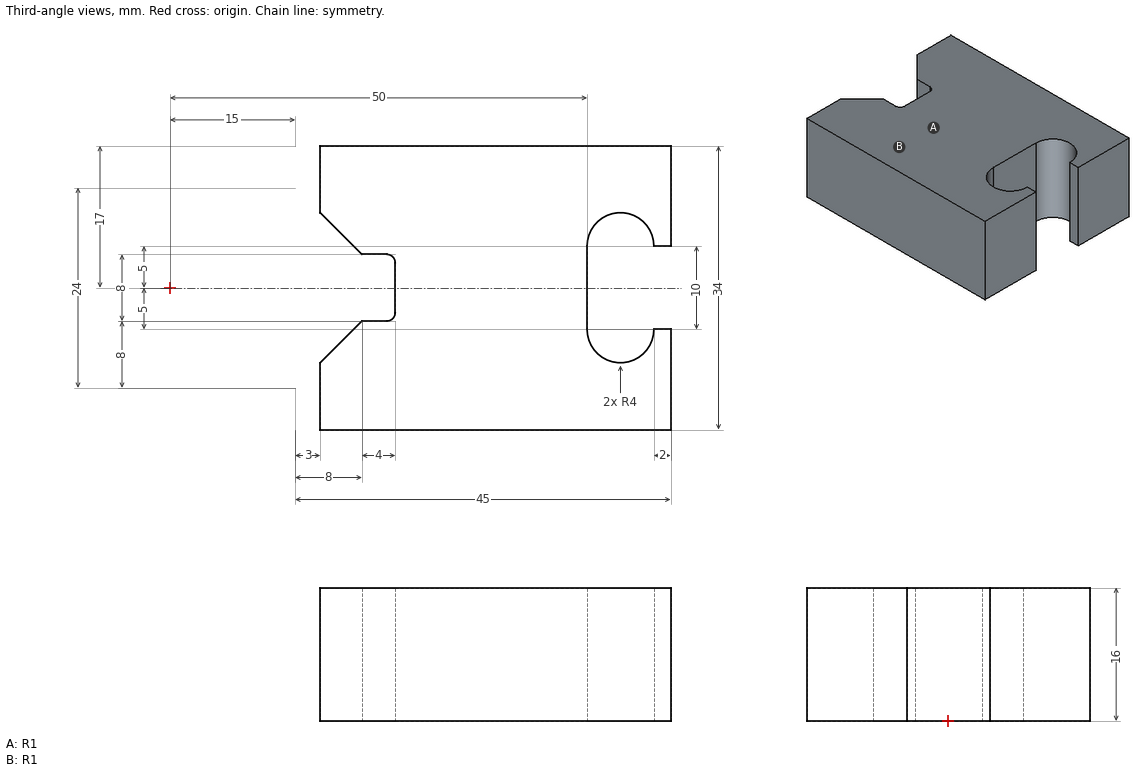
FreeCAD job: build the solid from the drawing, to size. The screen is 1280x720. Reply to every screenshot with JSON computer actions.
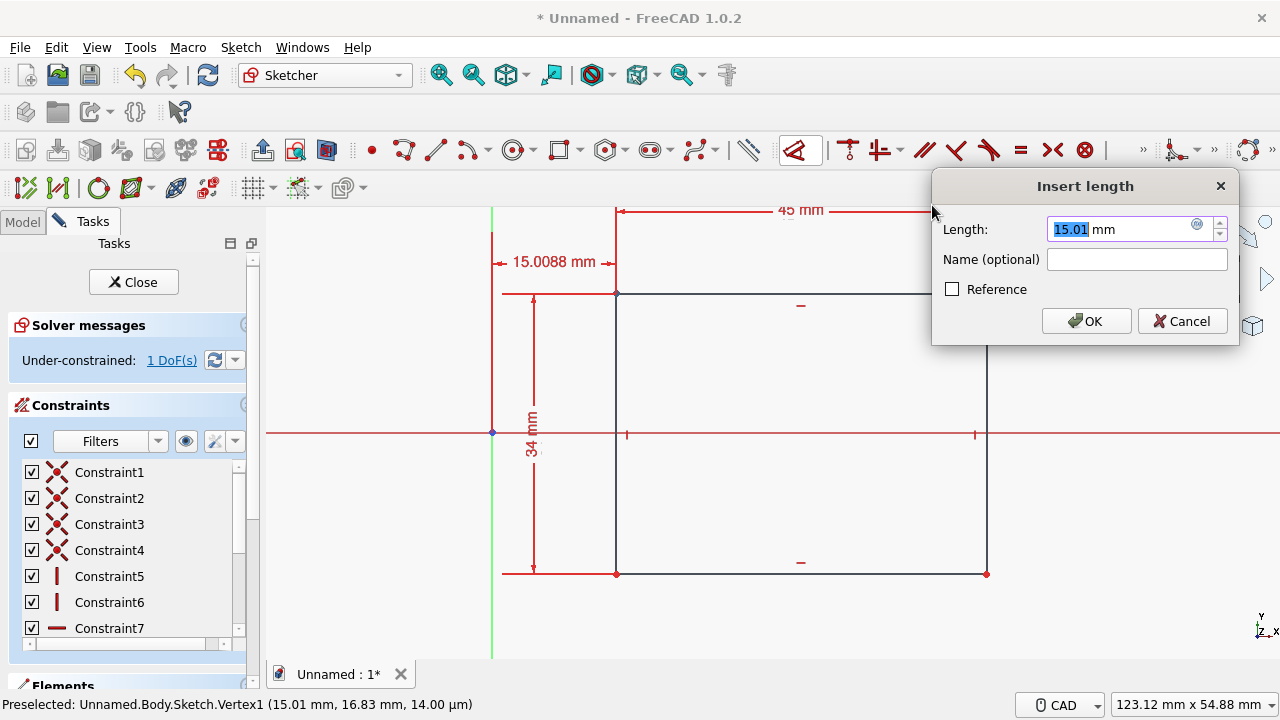
{"action": "type", "text": "15"}
{"action": "key", "text": "Return"}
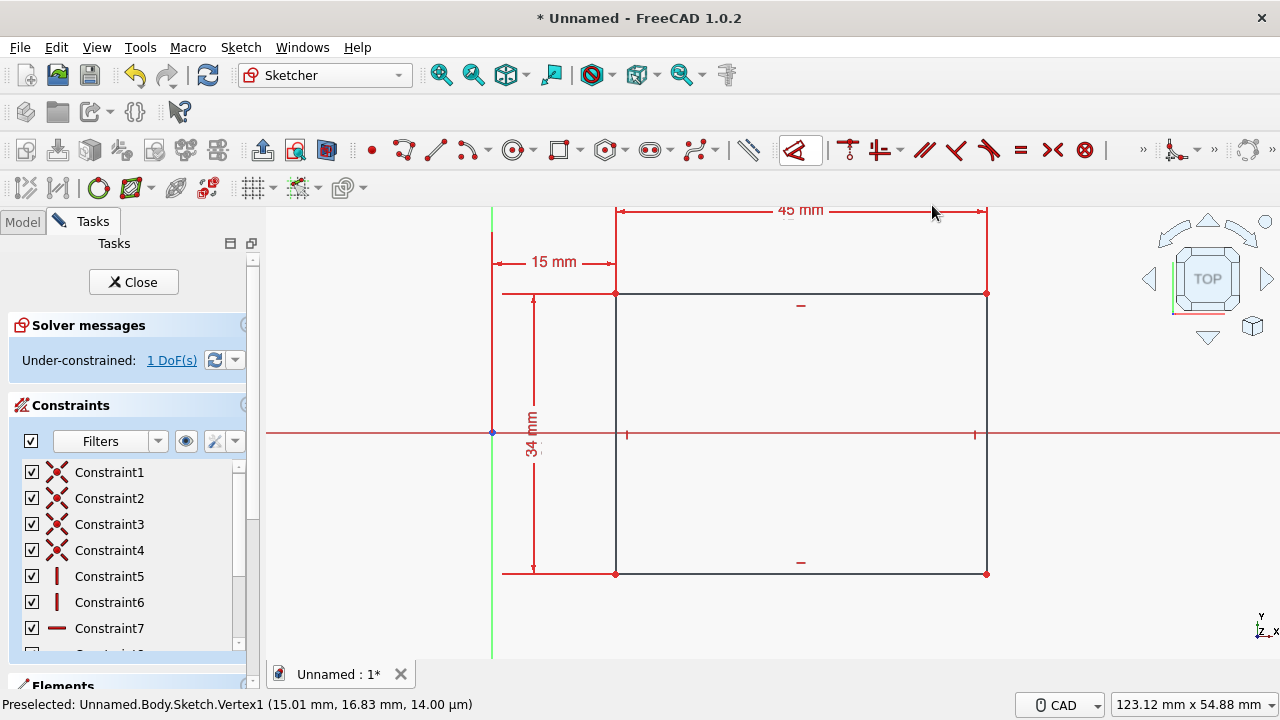
{"action": "left_click", "coordinate": [616, 294]}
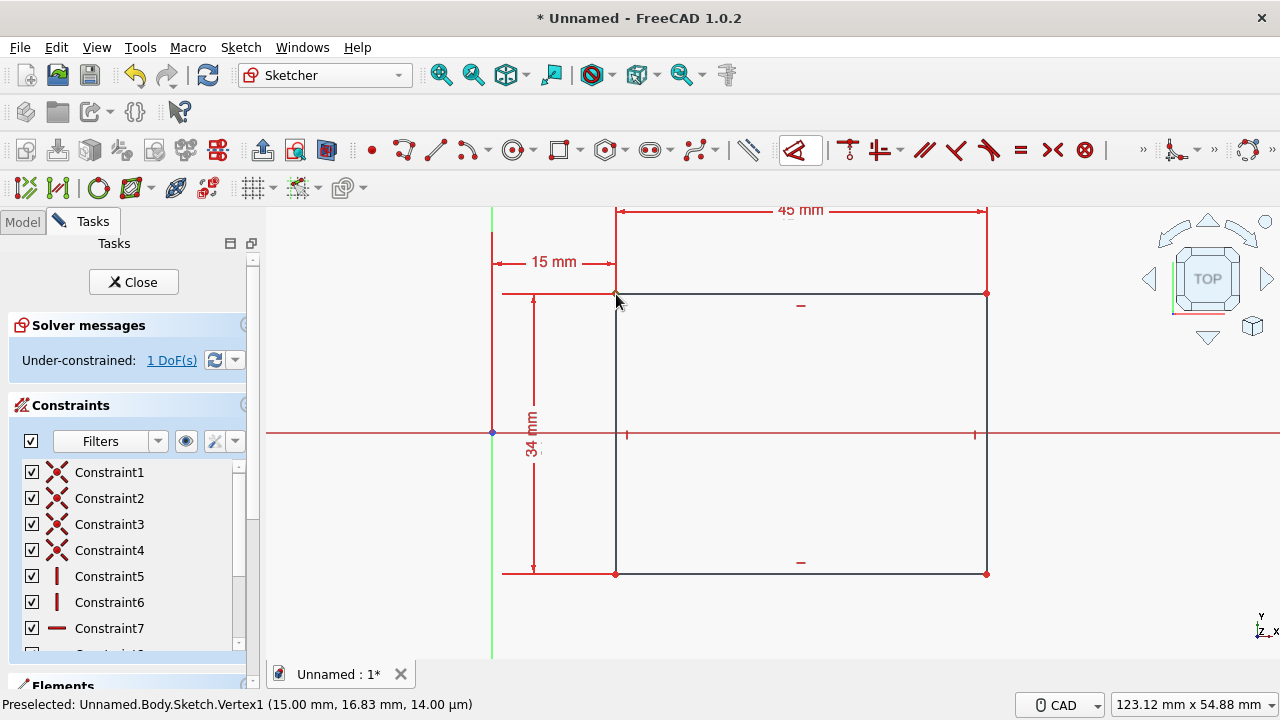
{"action": "left_click", "coordinate": [816, 150]}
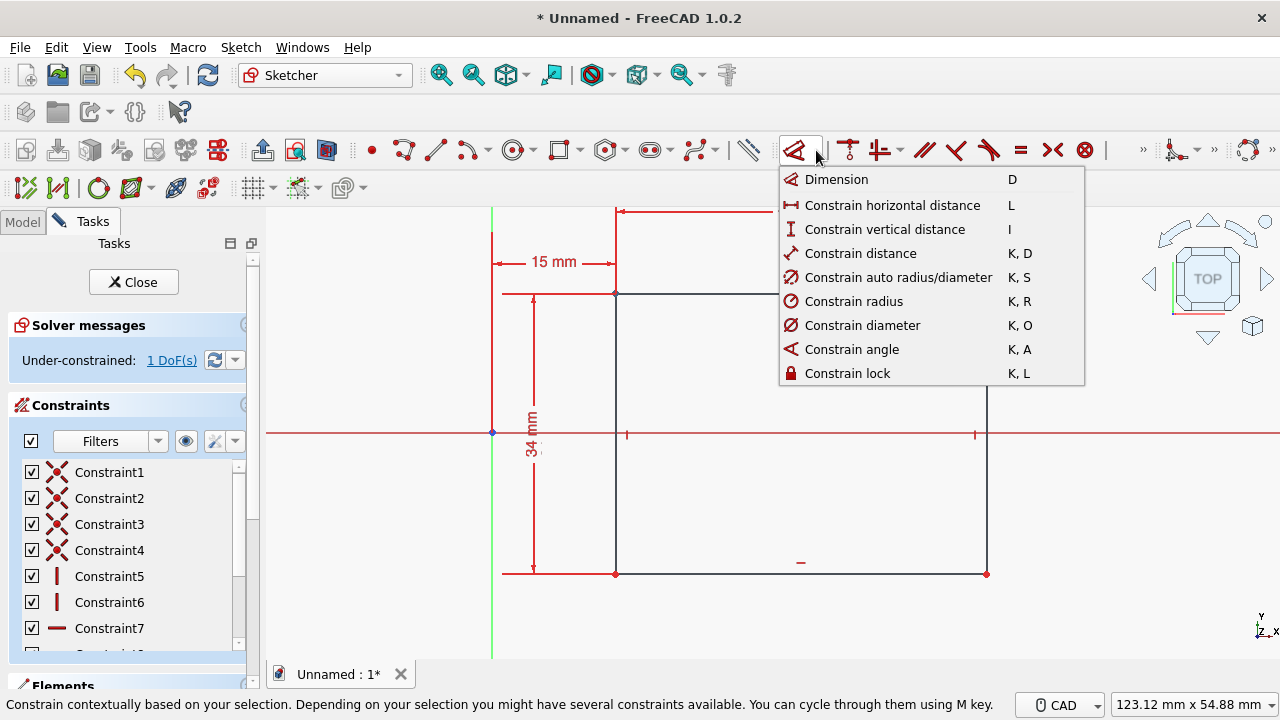
{"action": "left_click", "coordinate": [932, 229]}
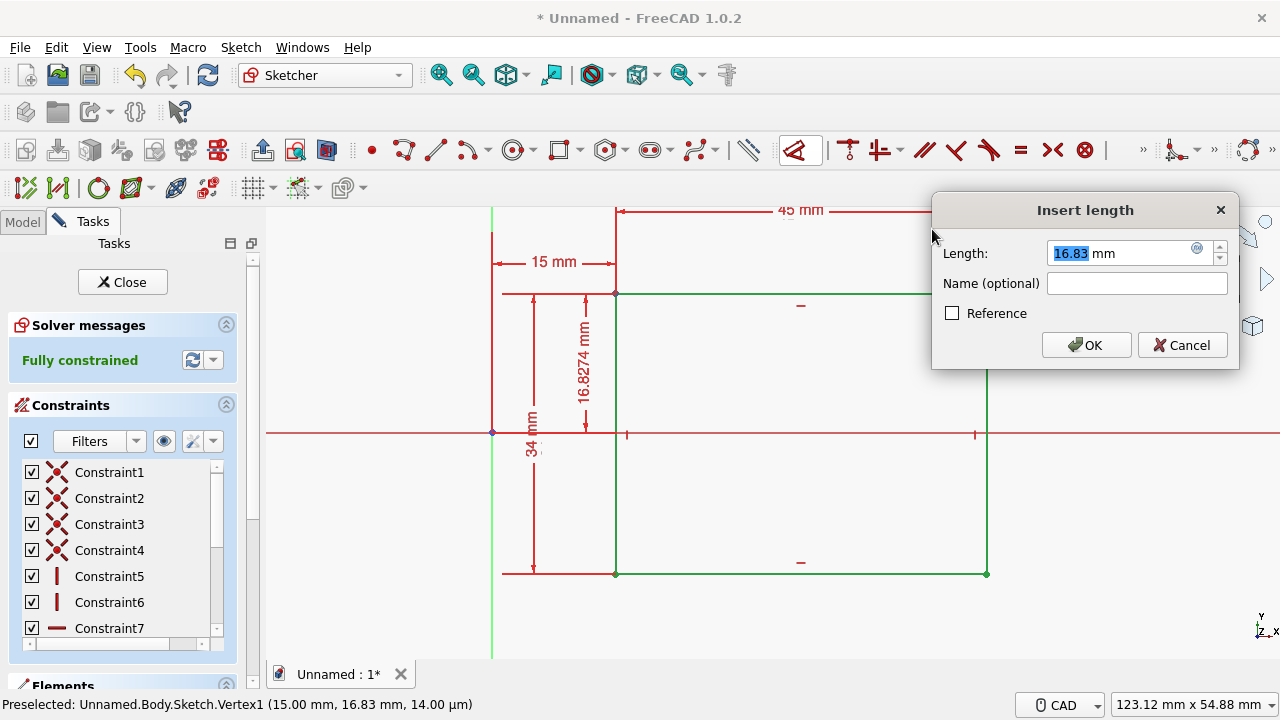
{"action": "type", "text": "17"}
{"action": "key", "text": "Return"}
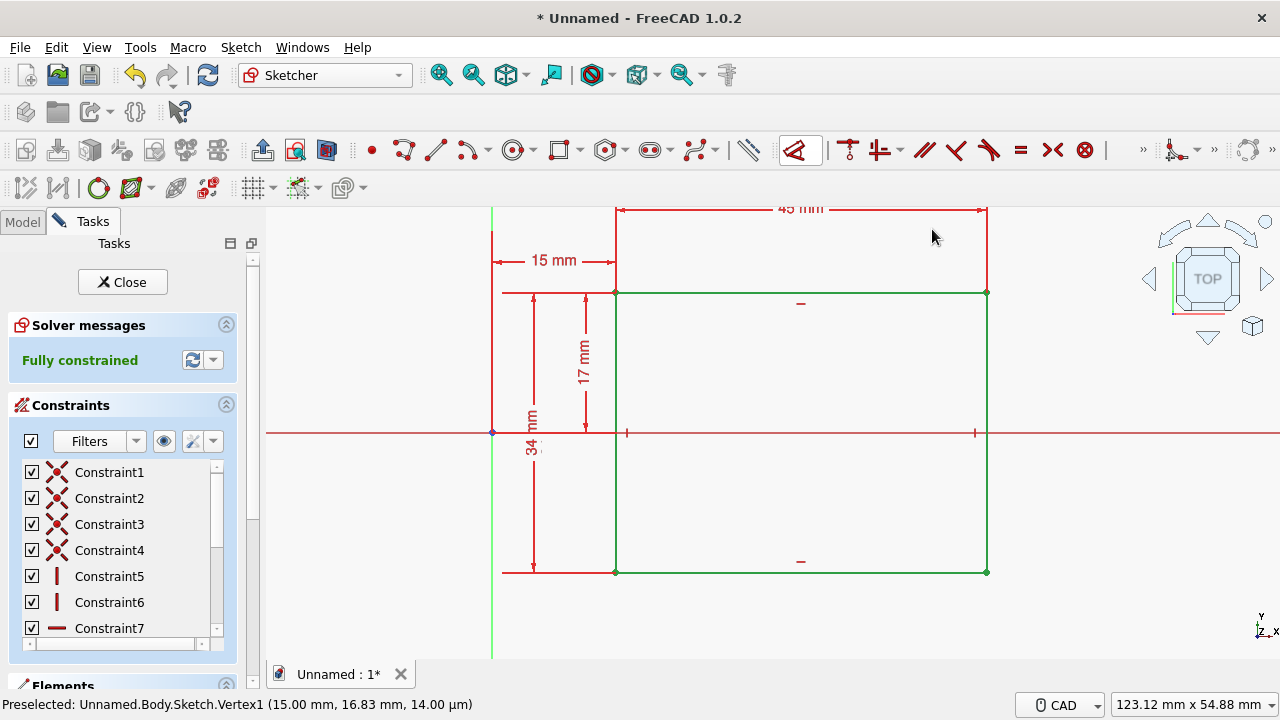
{"action": "left_click", "coordinate": [123, 282]}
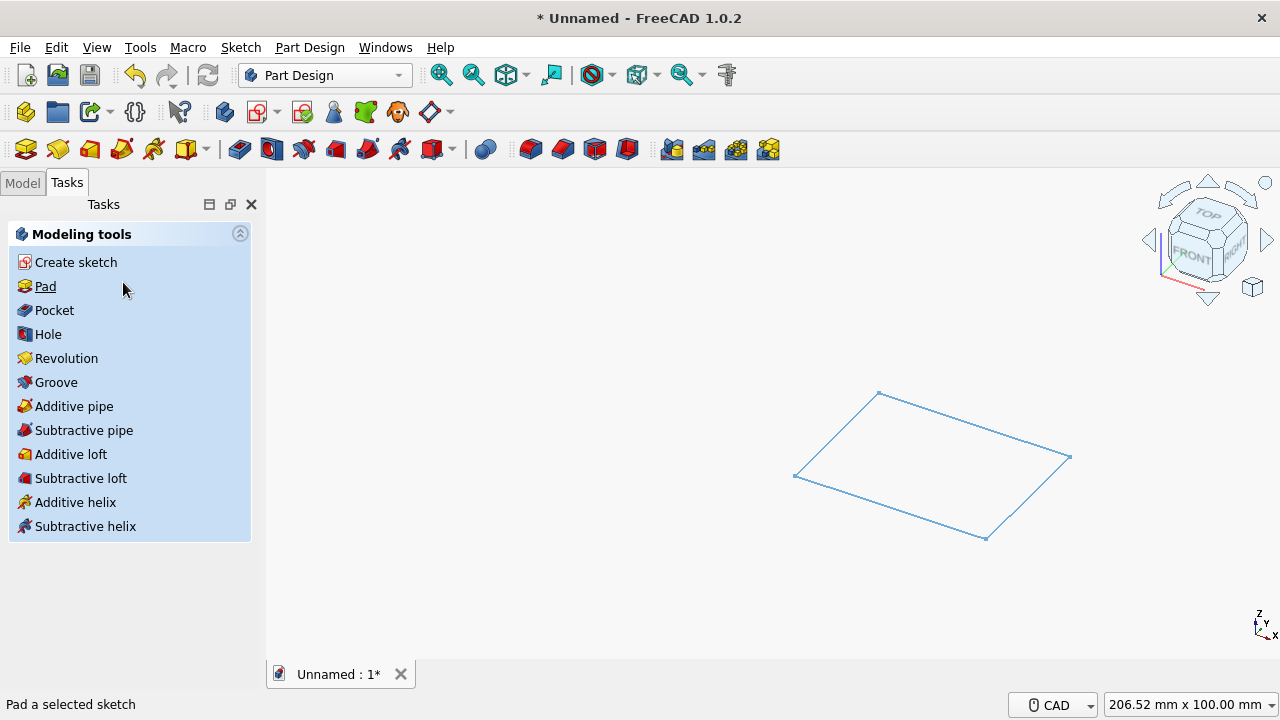
{"action": "left_click", "coordinate": [26, 150]}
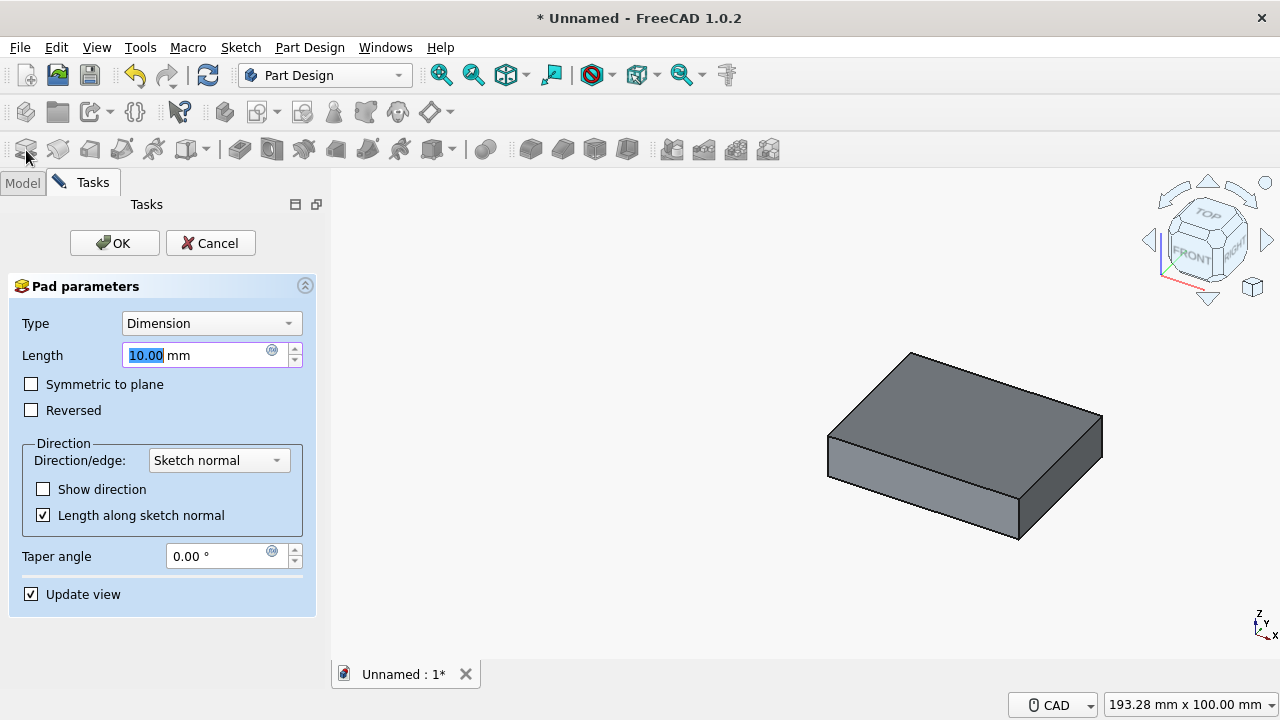
{"action": "type", "text": "16"}
{"action": "key", "text": "Tab"}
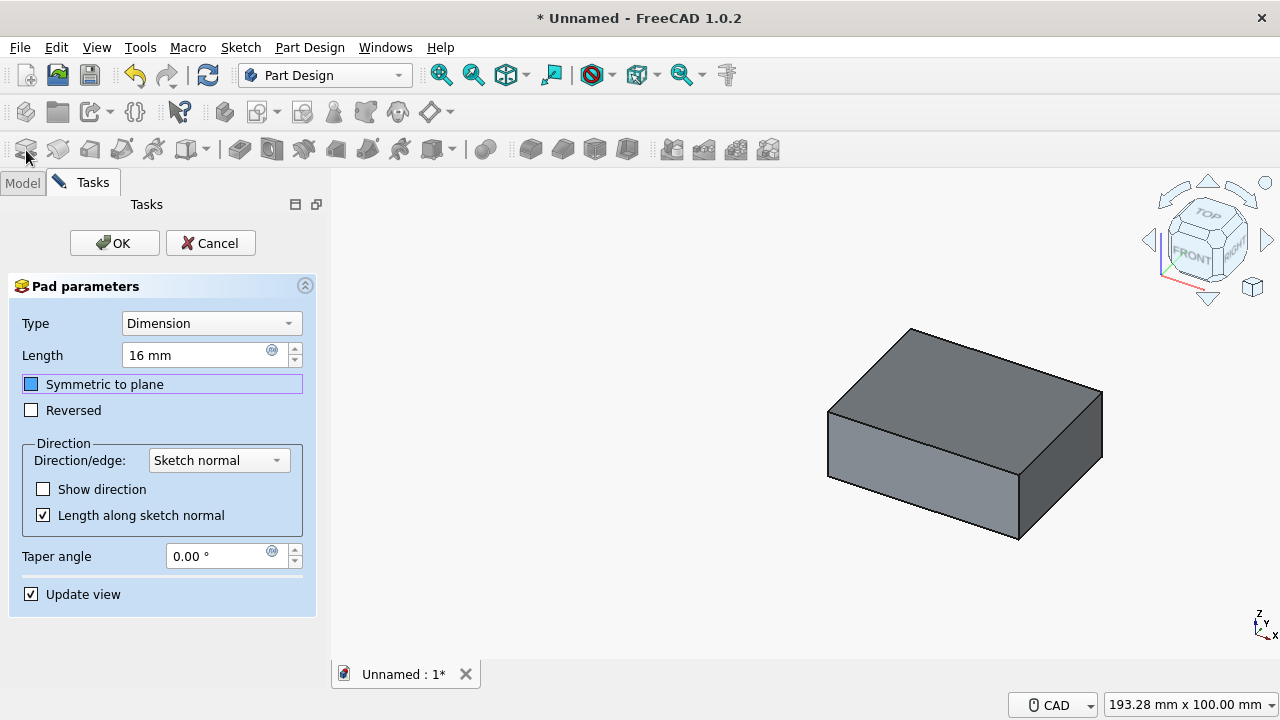
{"action": "left_click", "coordinate": [115, 243]}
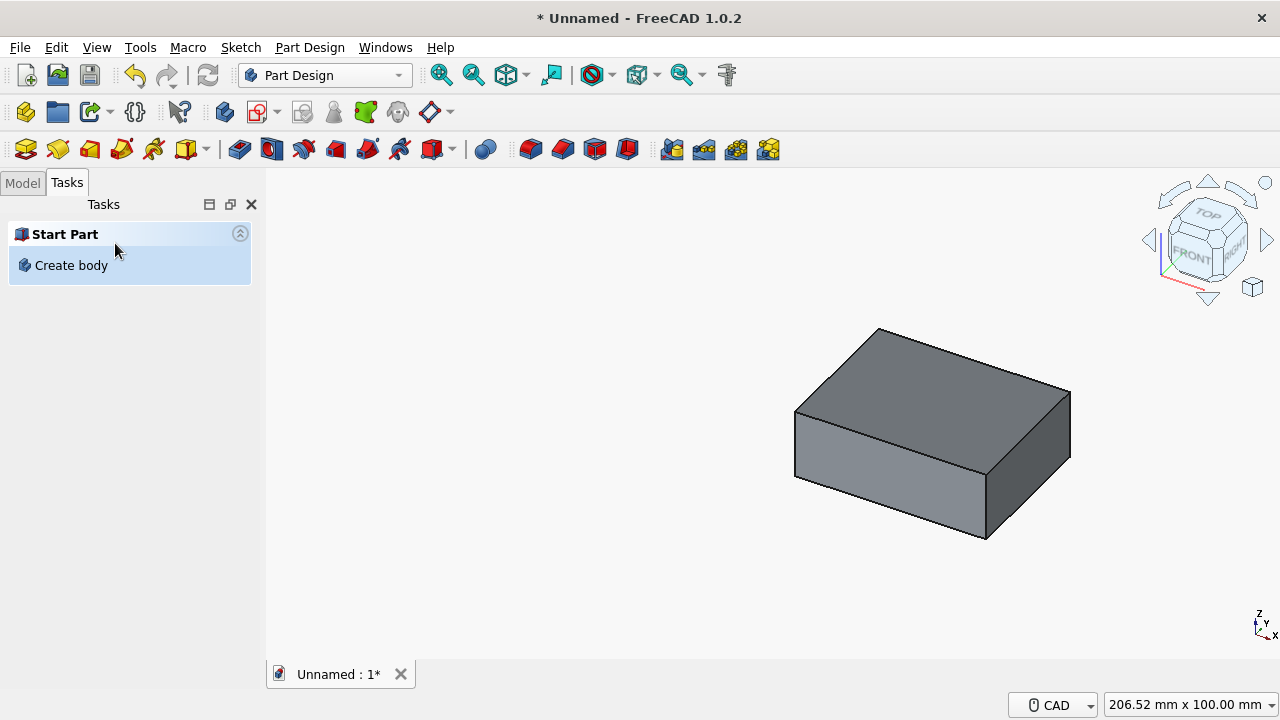
{"action": "left_click", "coordinate": [442, 76]}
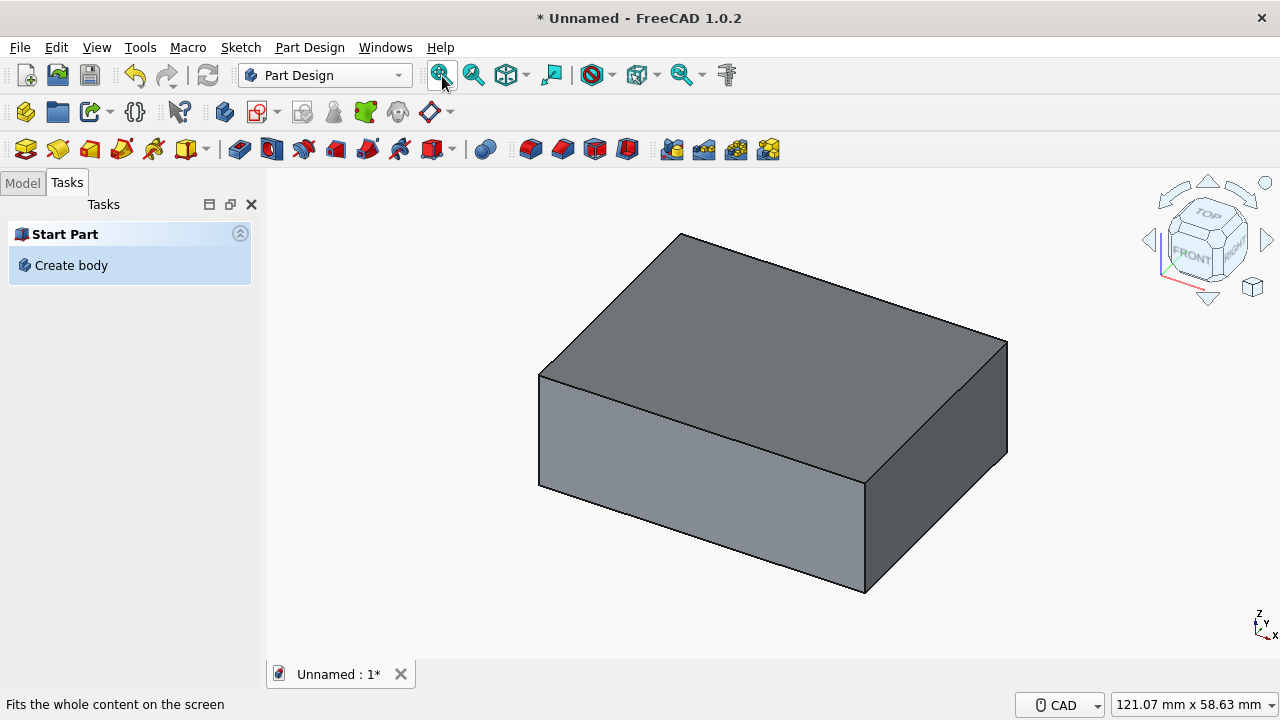
{"action": "left_click", "coordinate": [773, 358]}